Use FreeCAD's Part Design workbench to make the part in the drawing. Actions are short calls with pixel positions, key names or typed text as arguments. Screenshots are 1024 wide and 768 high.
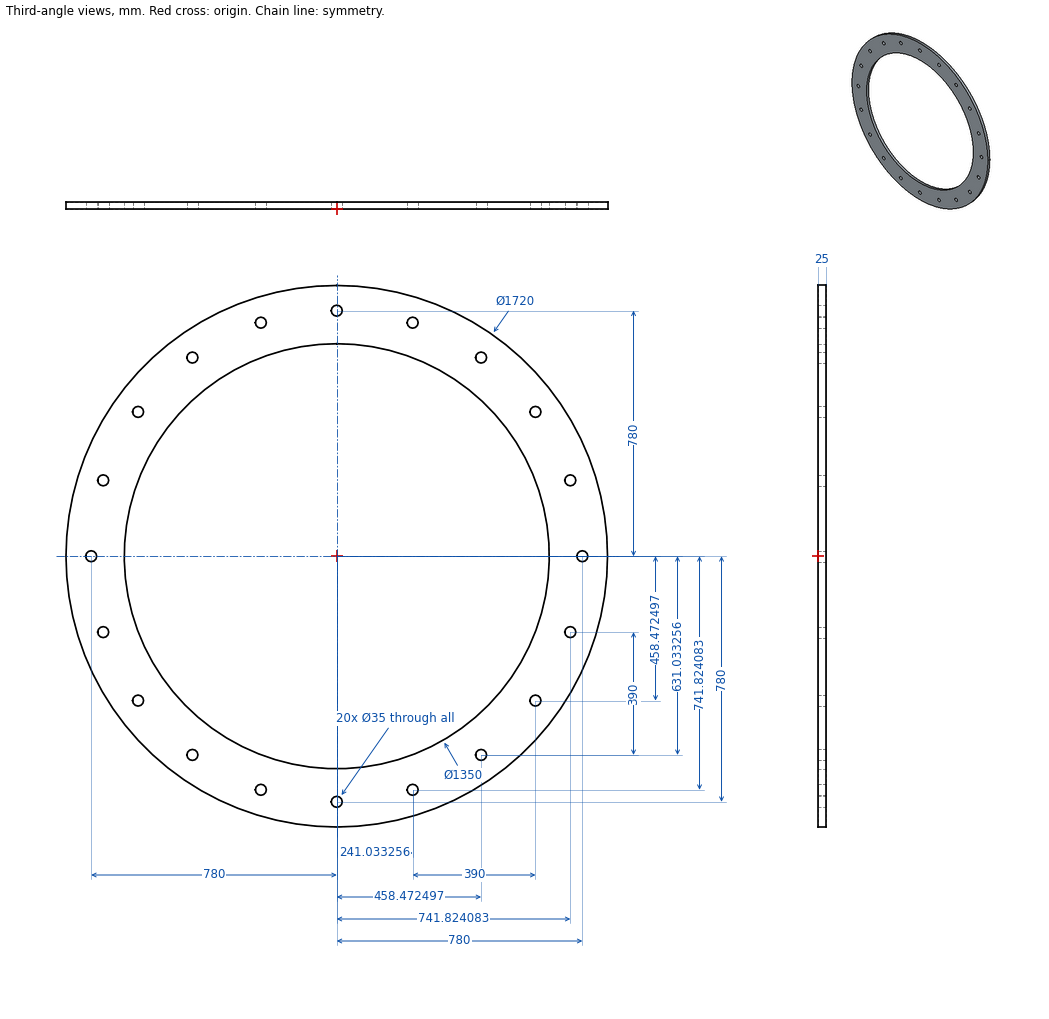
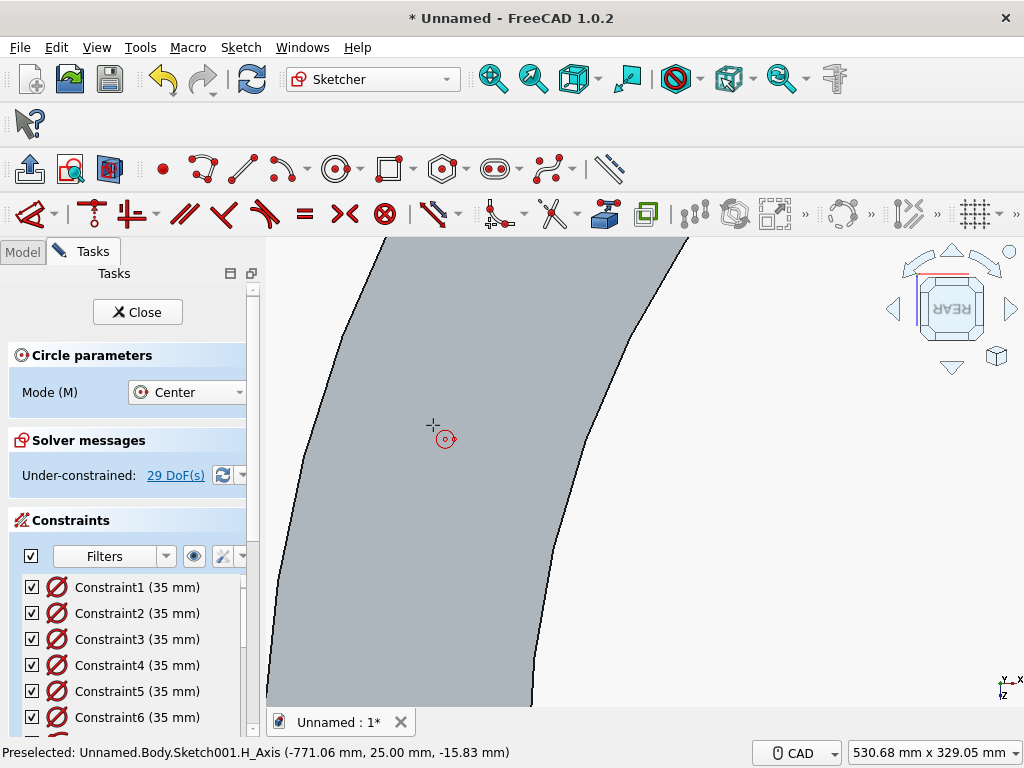
scroll(433, 425, down, 10)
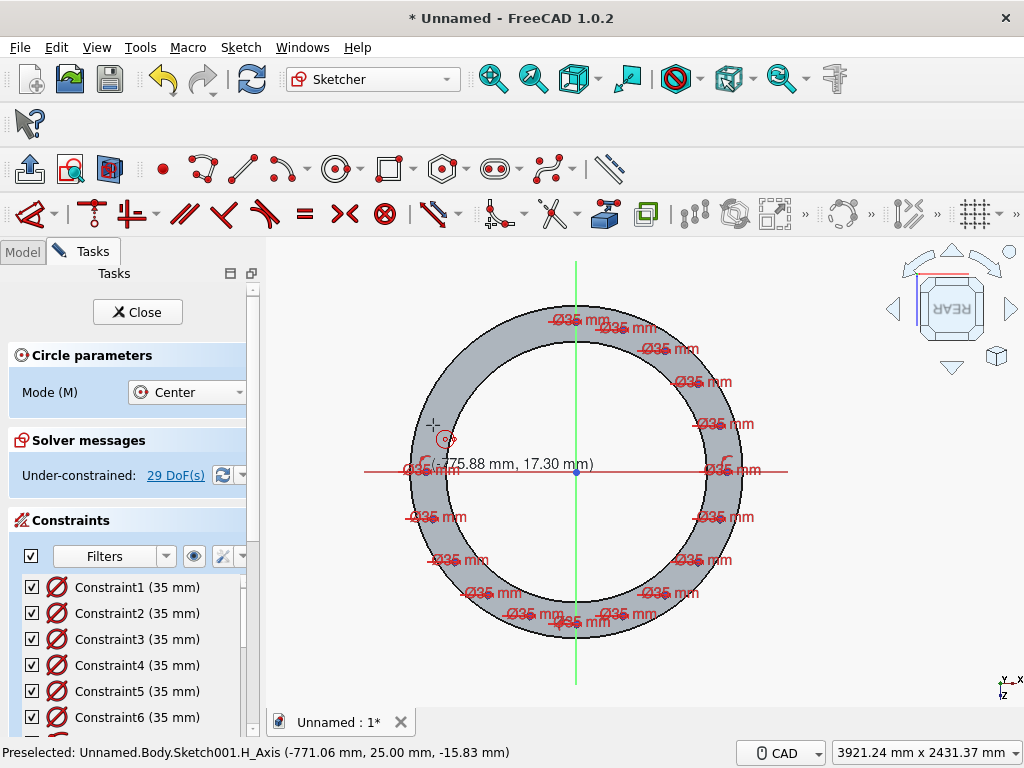
click(433, 425)
move(435, 423)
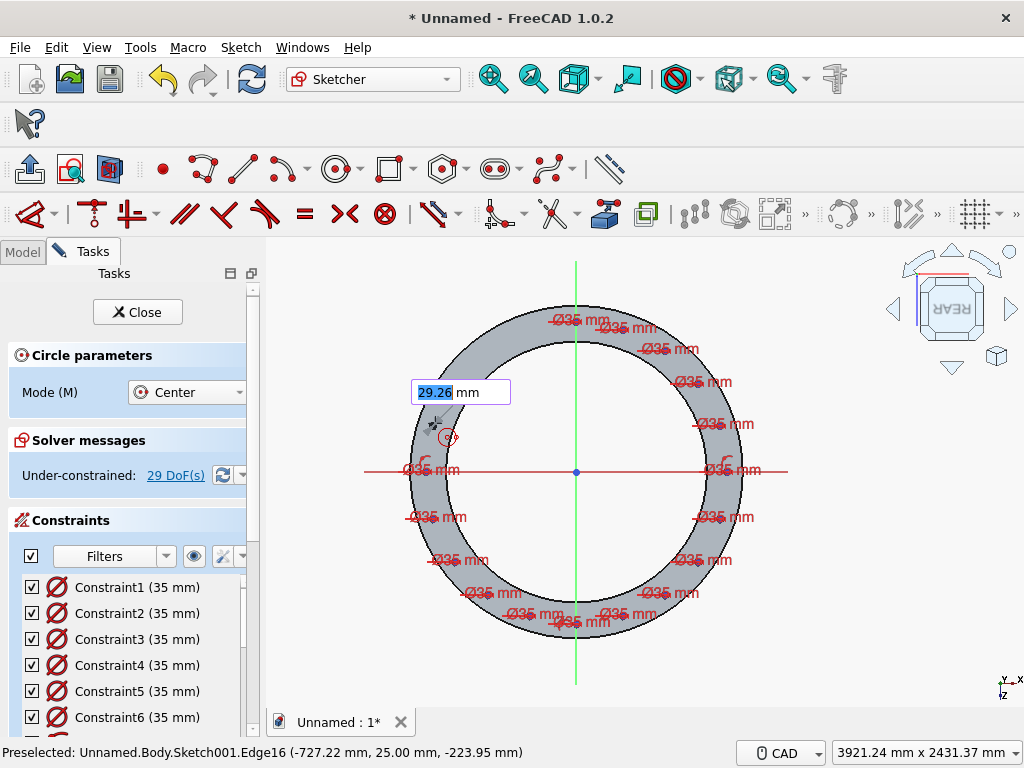
text(35)
key(Return)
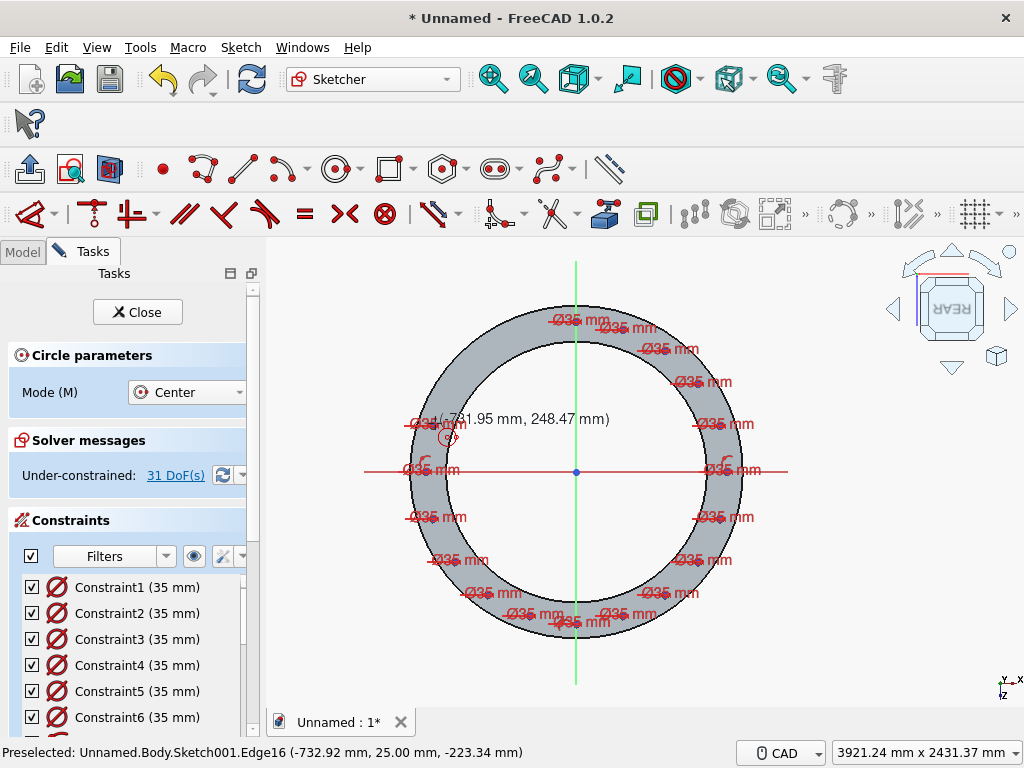
scroll(455, 383, up, 10)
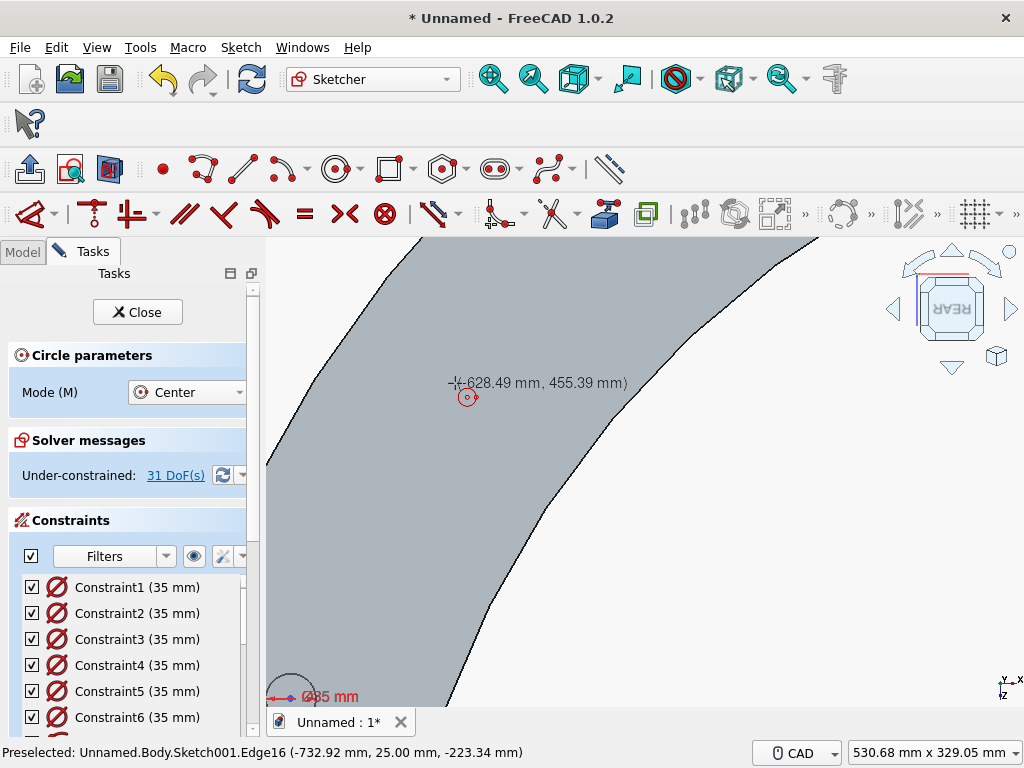
scroll(455, 383, down, 10)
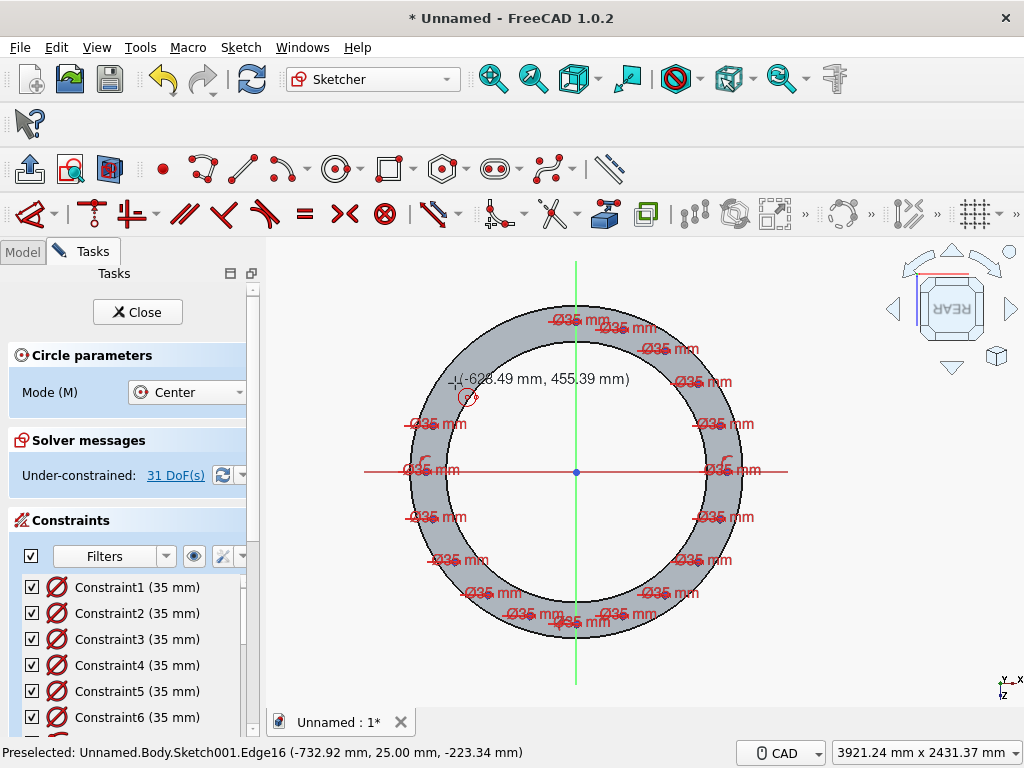
click(455, 383)
move(457, 381)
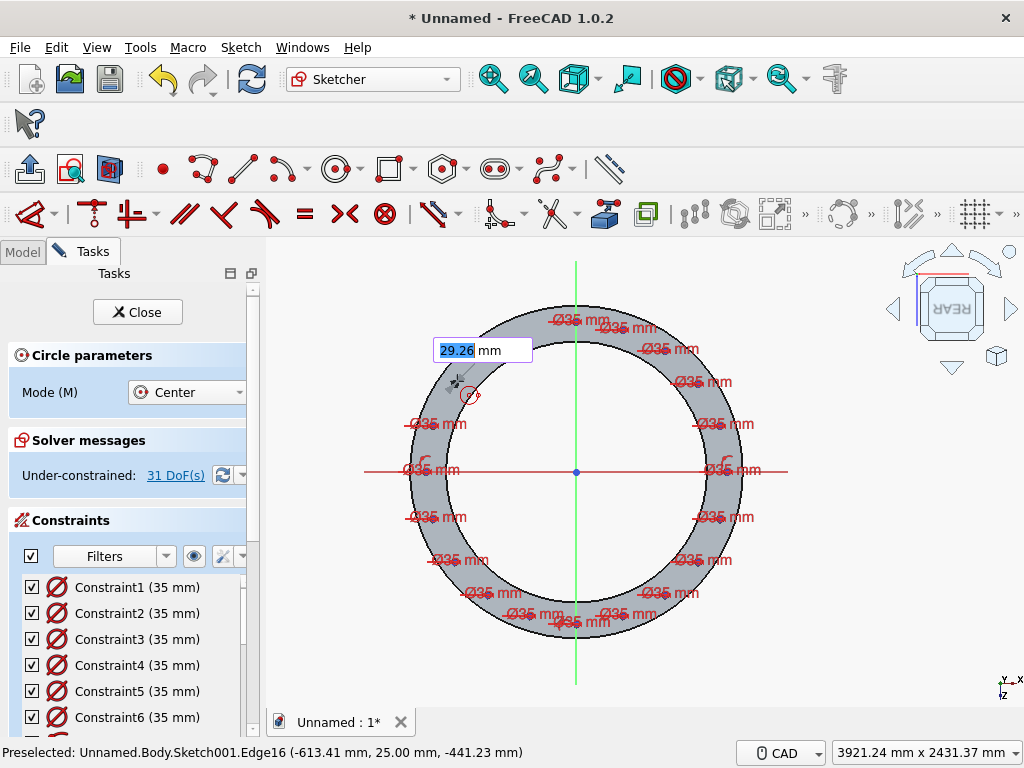
text(35)
key(Return)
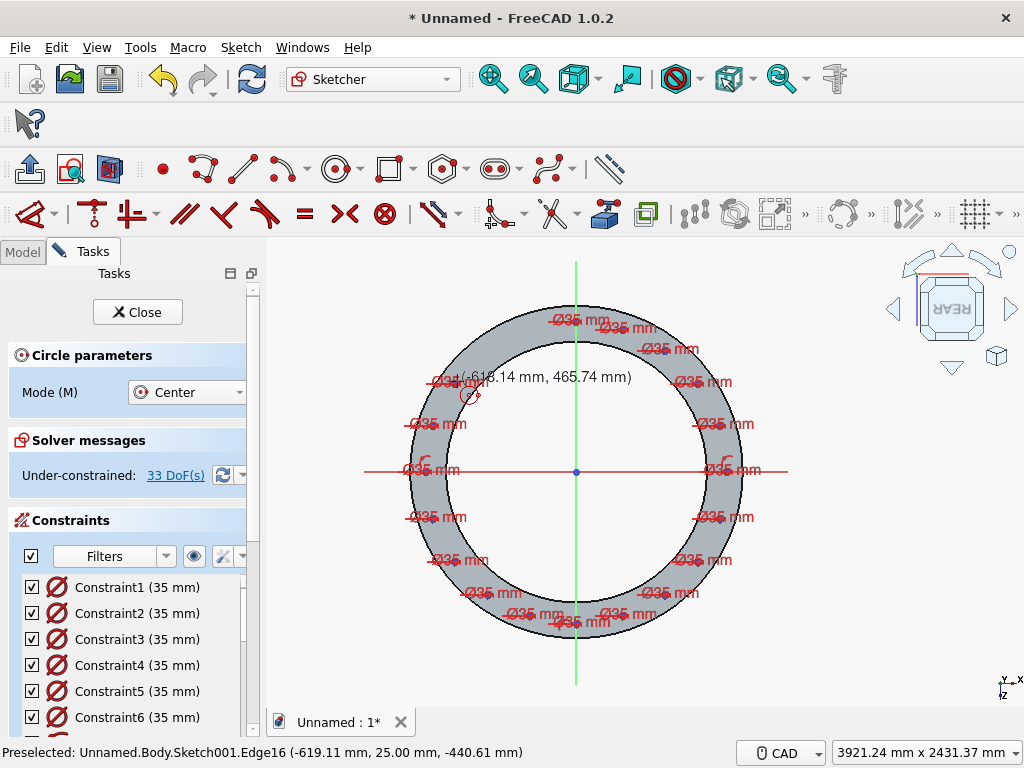
scroll(488, 350, up, 10)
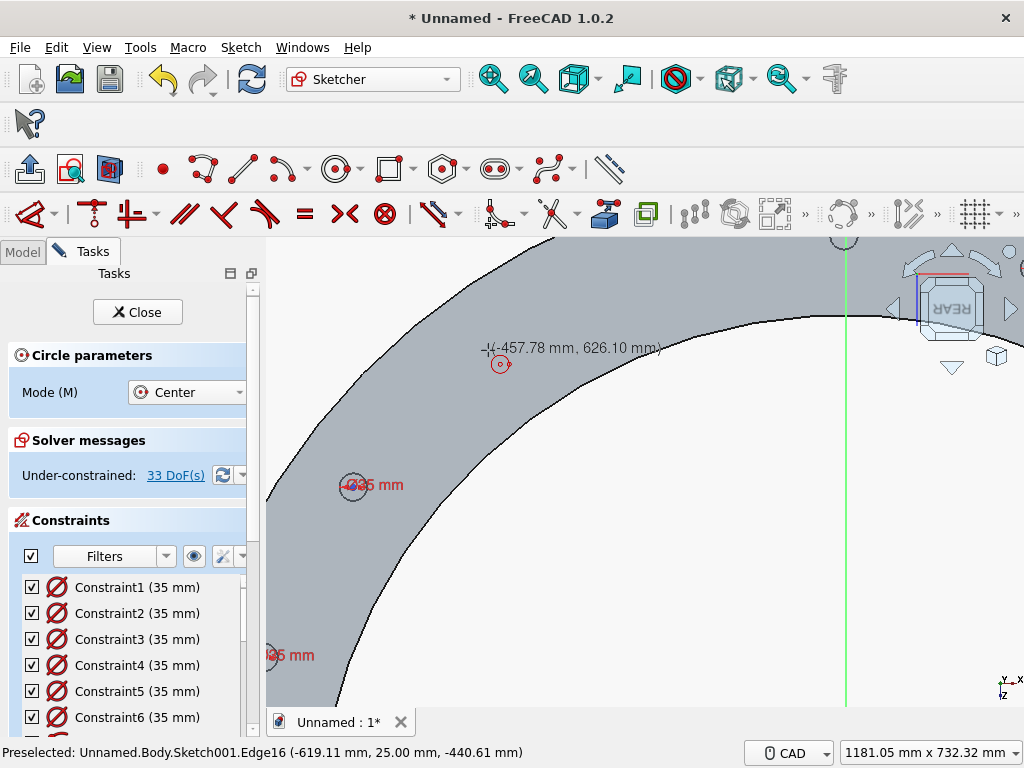
scroll(488, 350, down, 10)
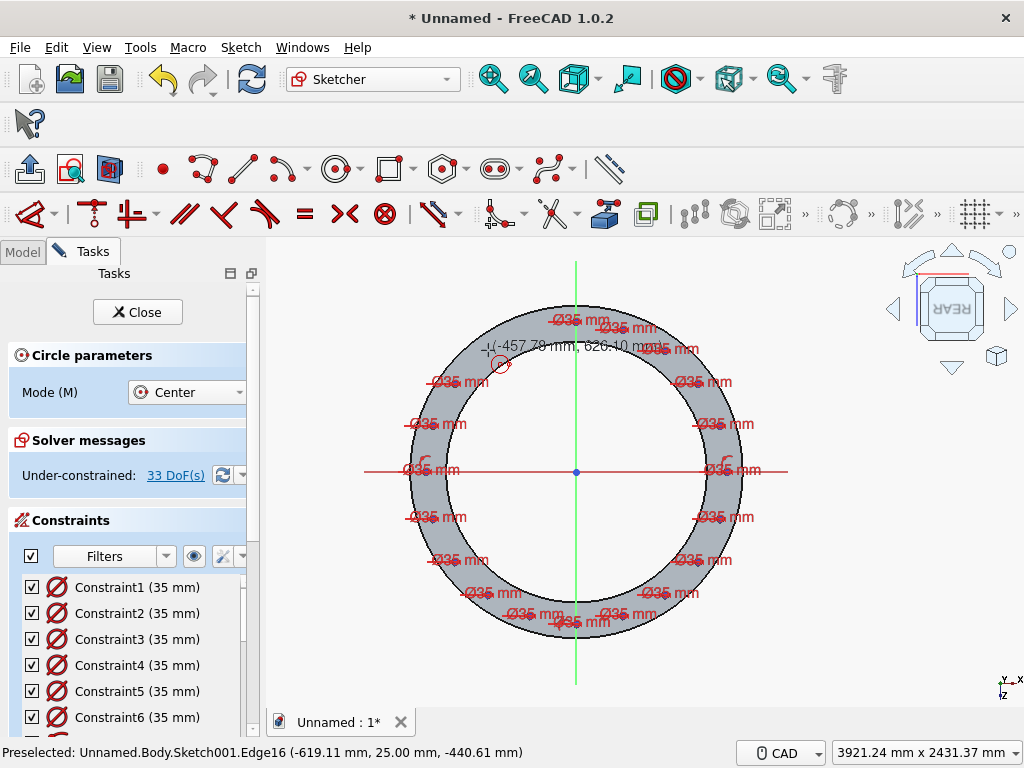
click(488, 350)
move(490, 348)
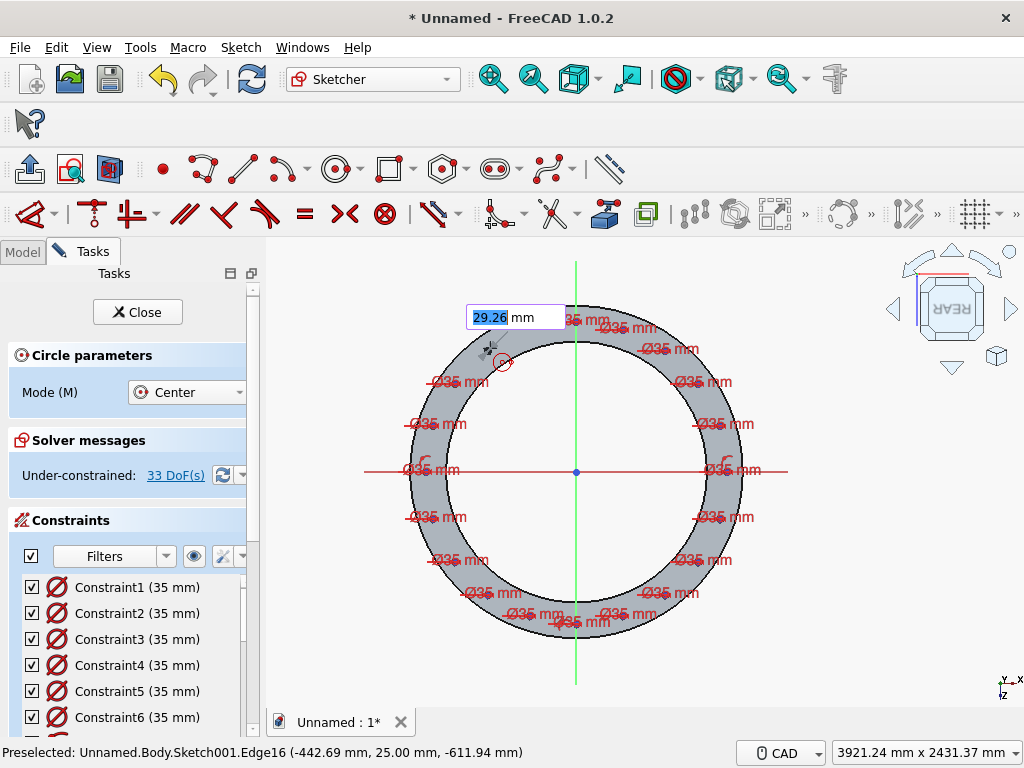
text(35)
key(Return)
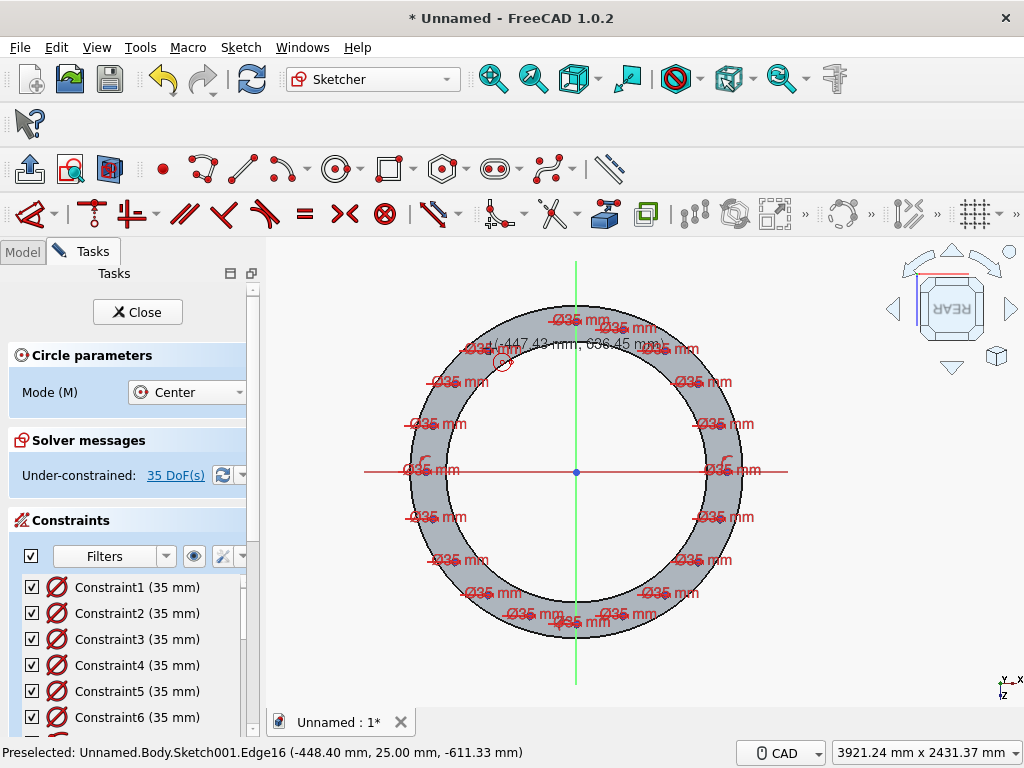
scroll(530, 329, up, 10)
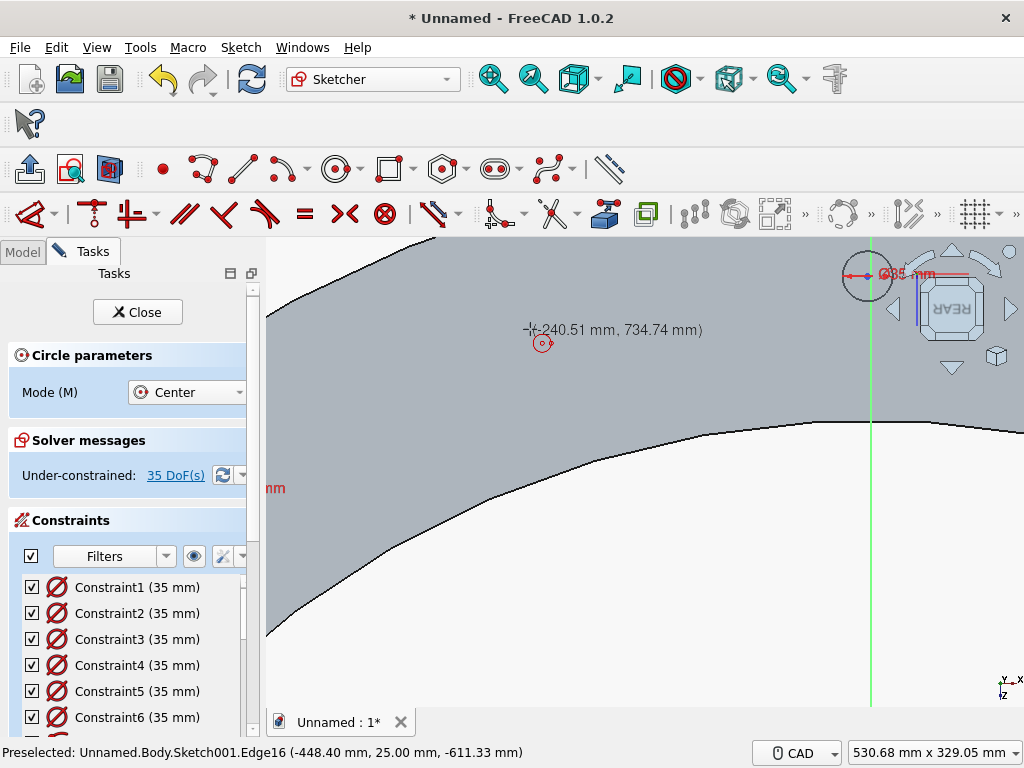
scroll(530, 329, down, 10)